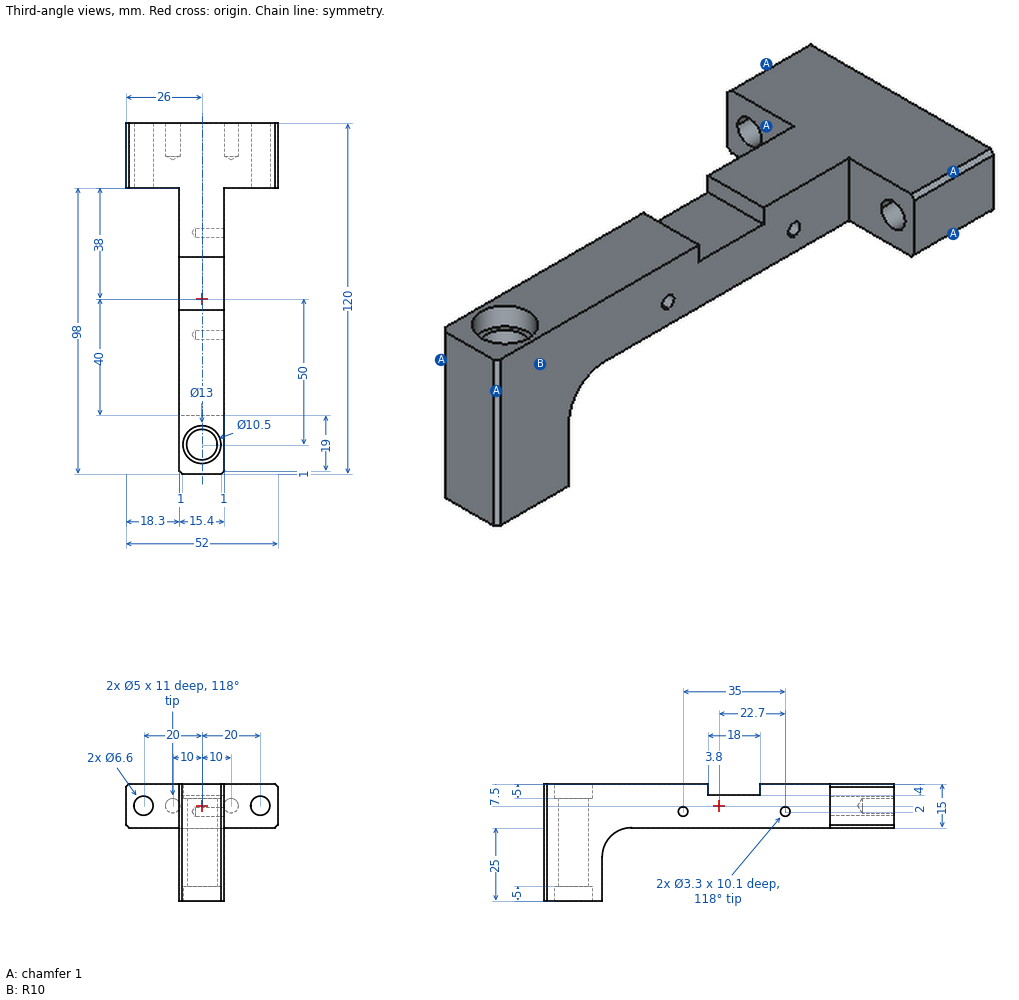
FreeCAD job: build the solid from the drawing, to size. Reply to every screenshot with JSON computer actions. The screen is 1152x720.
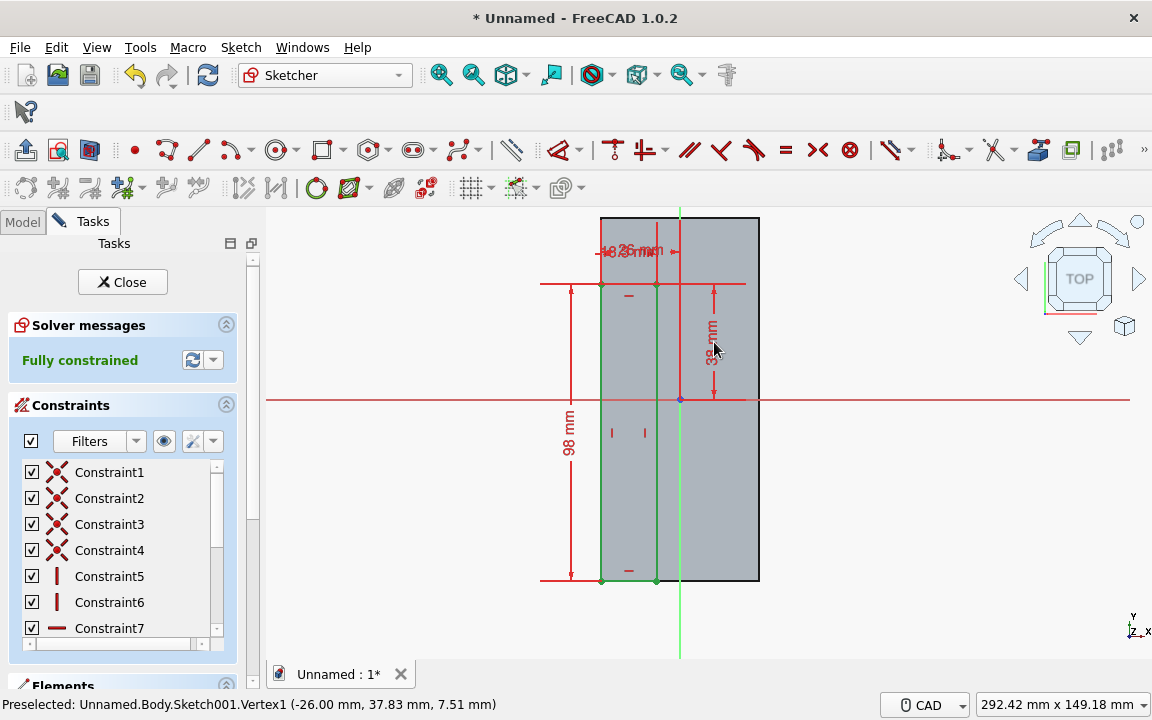
{"action": "left_click", "coordinate": [123, 282]}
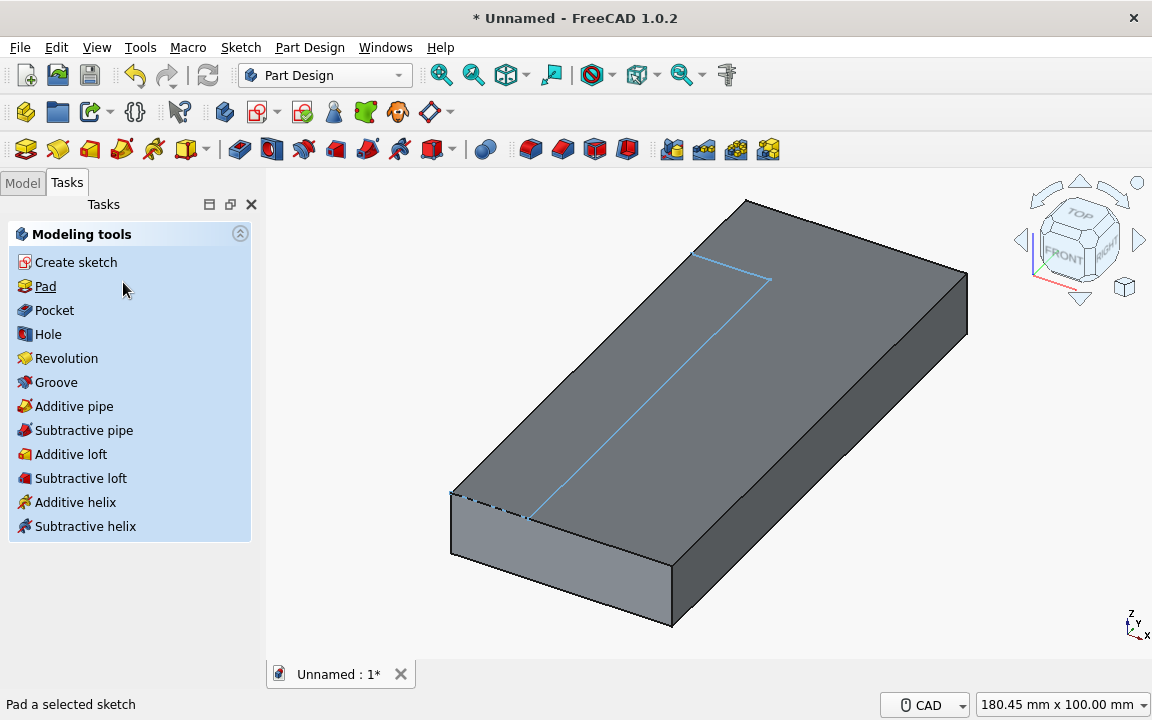
{"action": "left_click", "coordinate": [240, 150]}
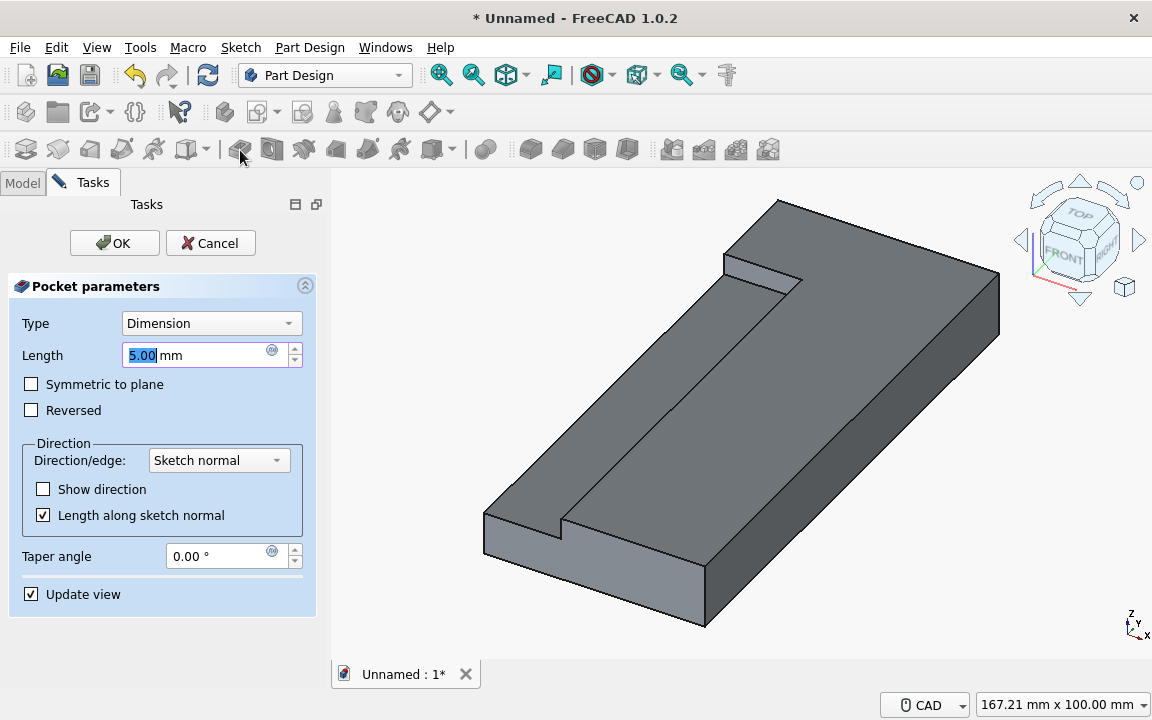
{"action": "left_click", "coordinate": [212, 324]}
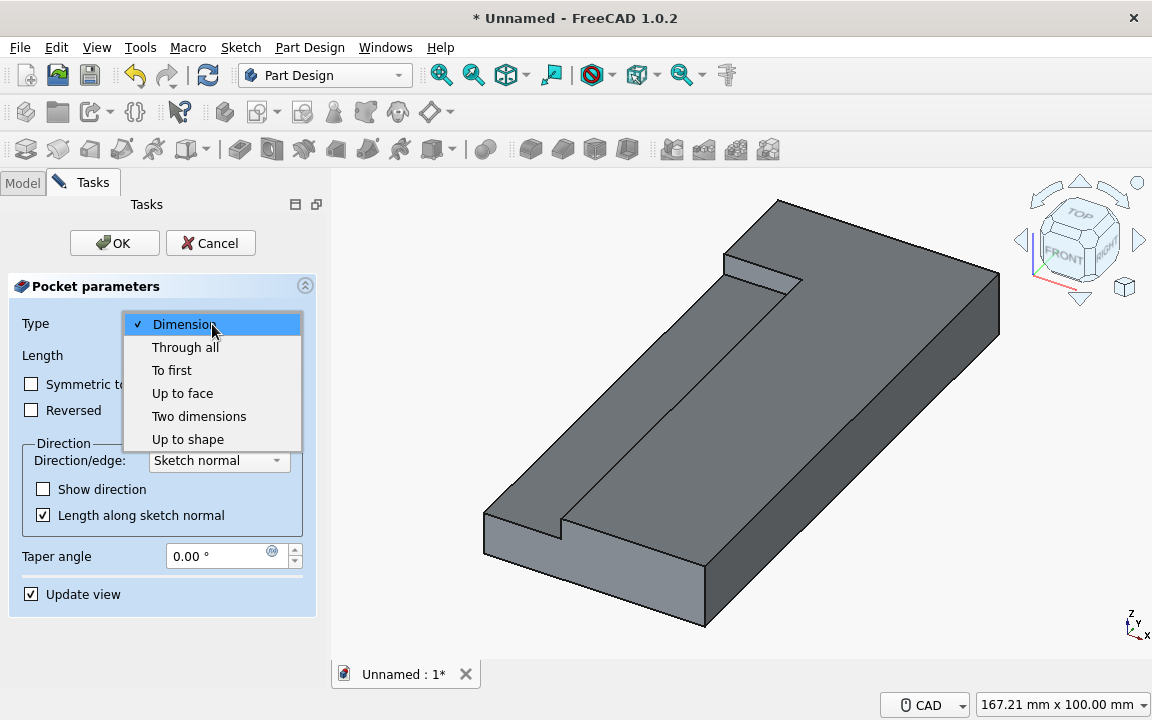
{"action": "left_click", "coordinate": [212, 348]}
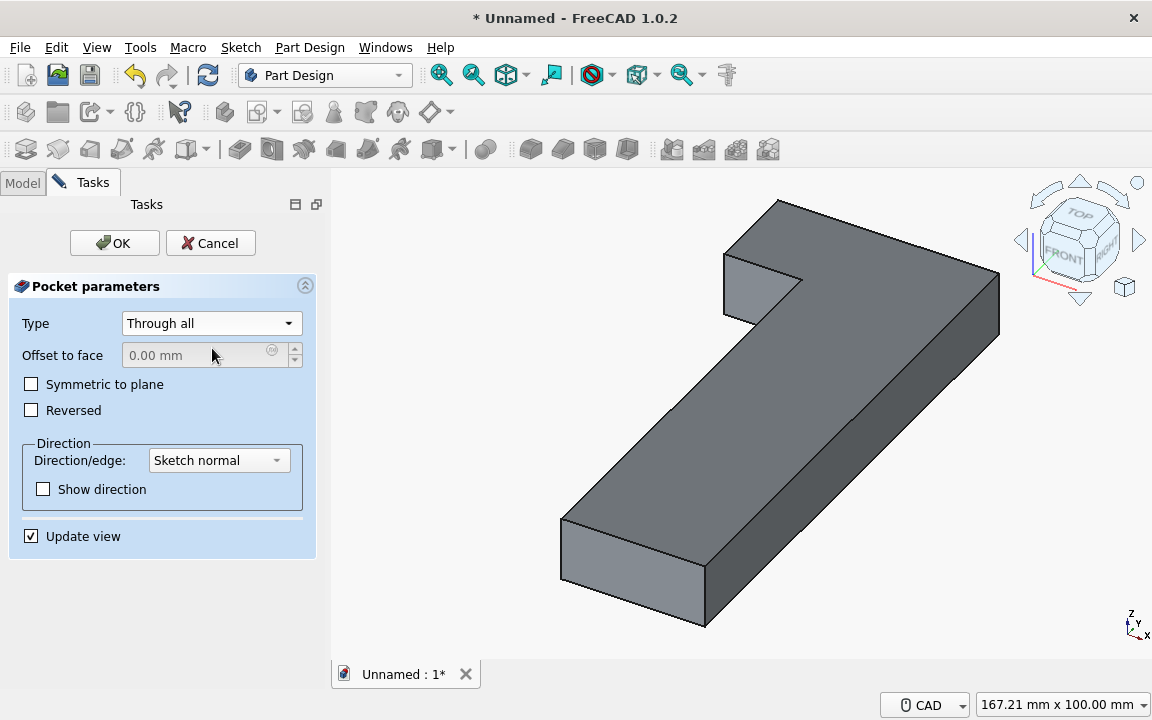
{"action": "left_click", "coordinate": [115, 243]}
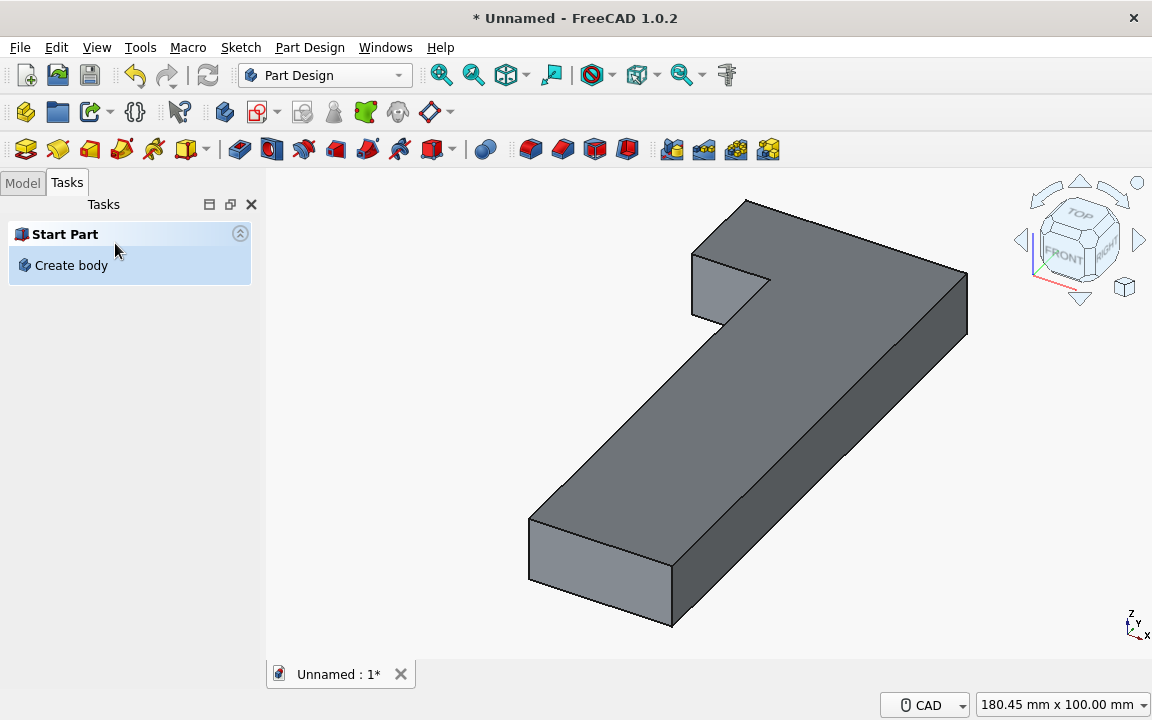
{"action": "left_click", "coordinate": [23, 182]}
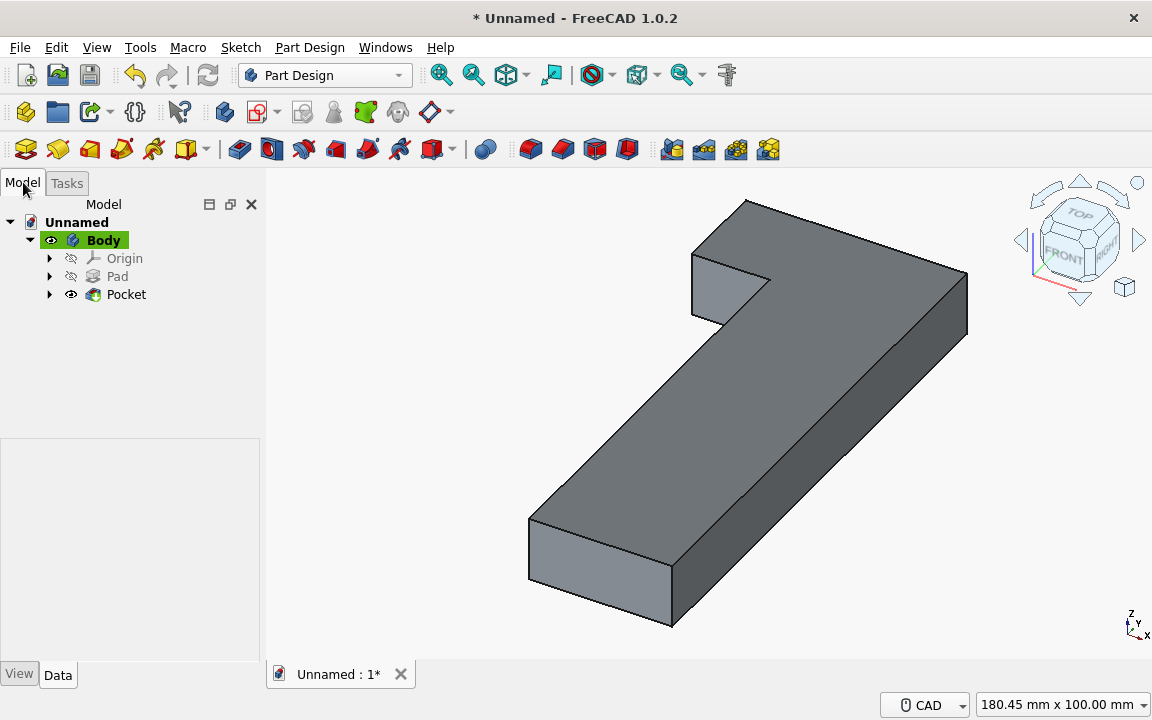
{"action": "left_click", "coordinate": [116, 294]}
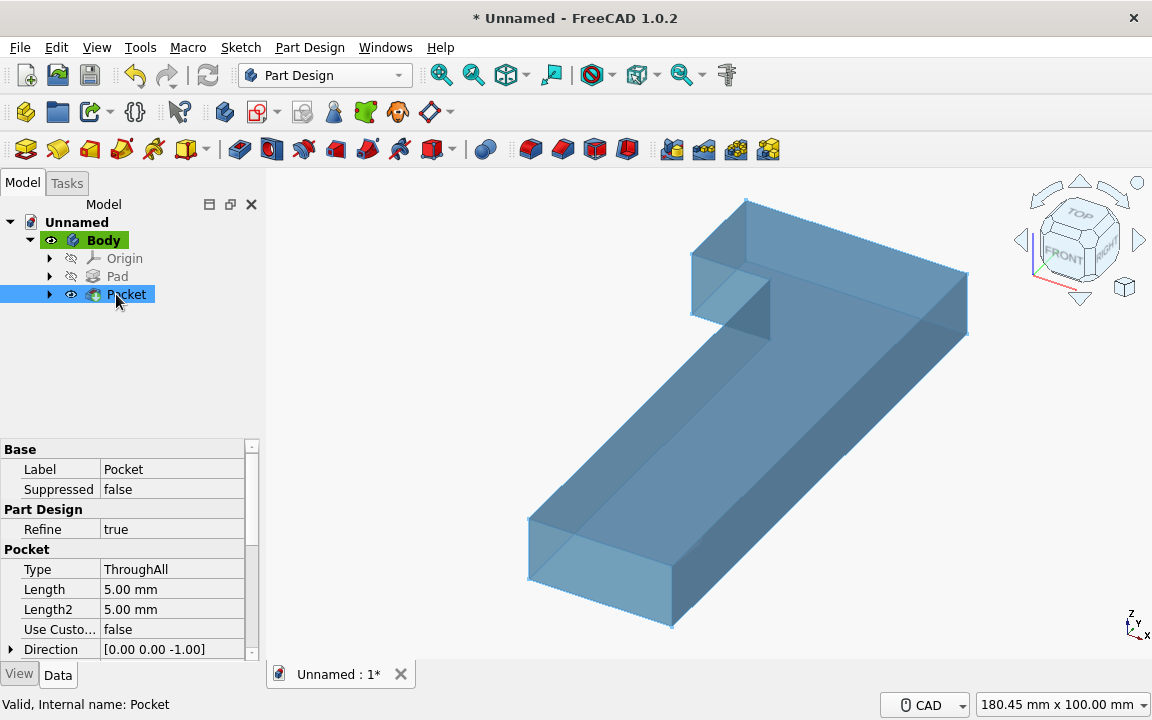
{"action": "left_click", "coordinate": [672, 150]}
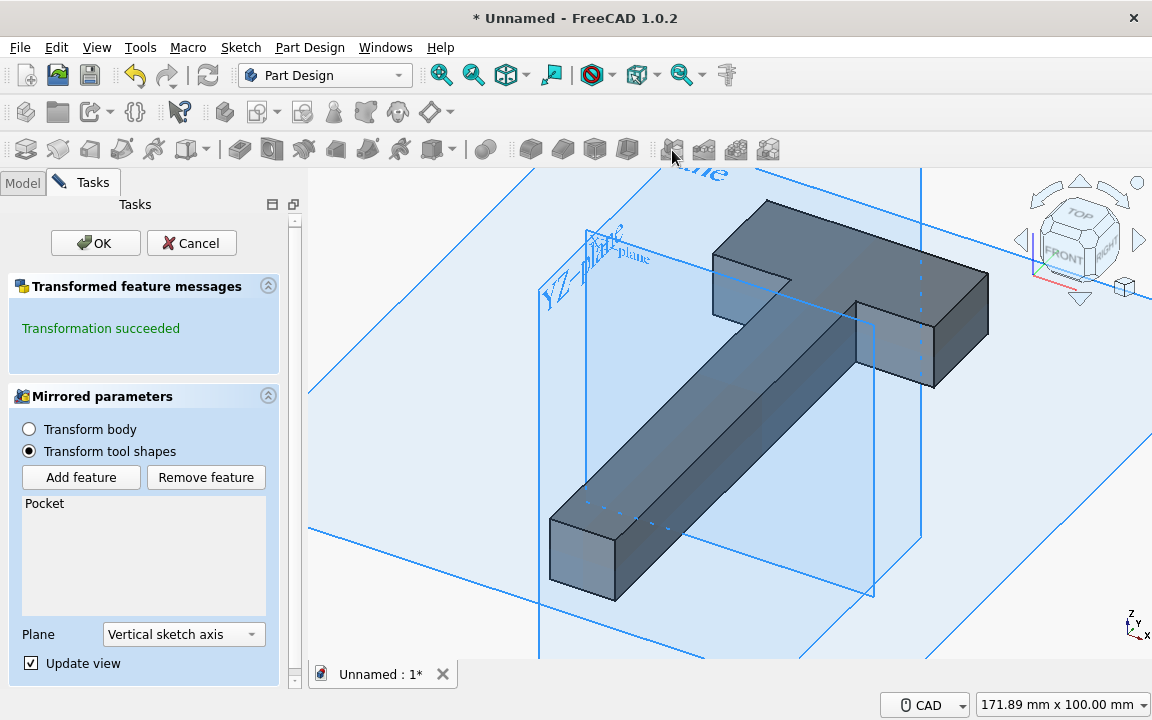
{"action": "left_click", "coordinate": [184, 634]}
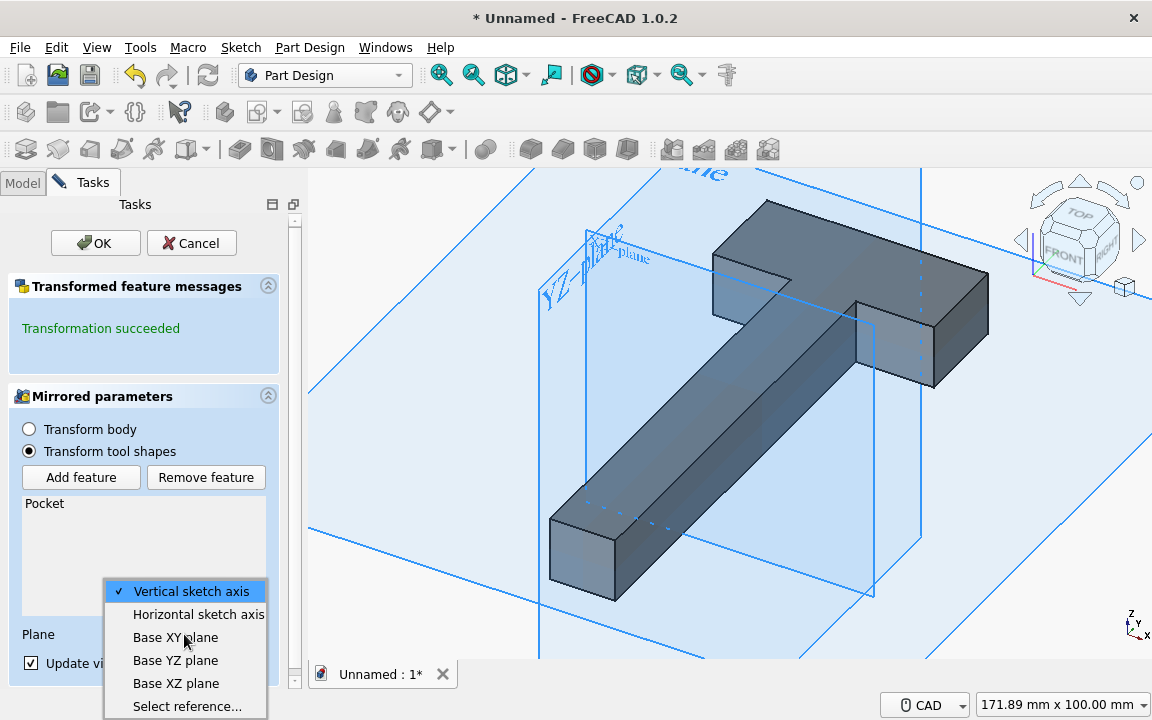
{"action": "left_click", "coordinate": [184, 660]}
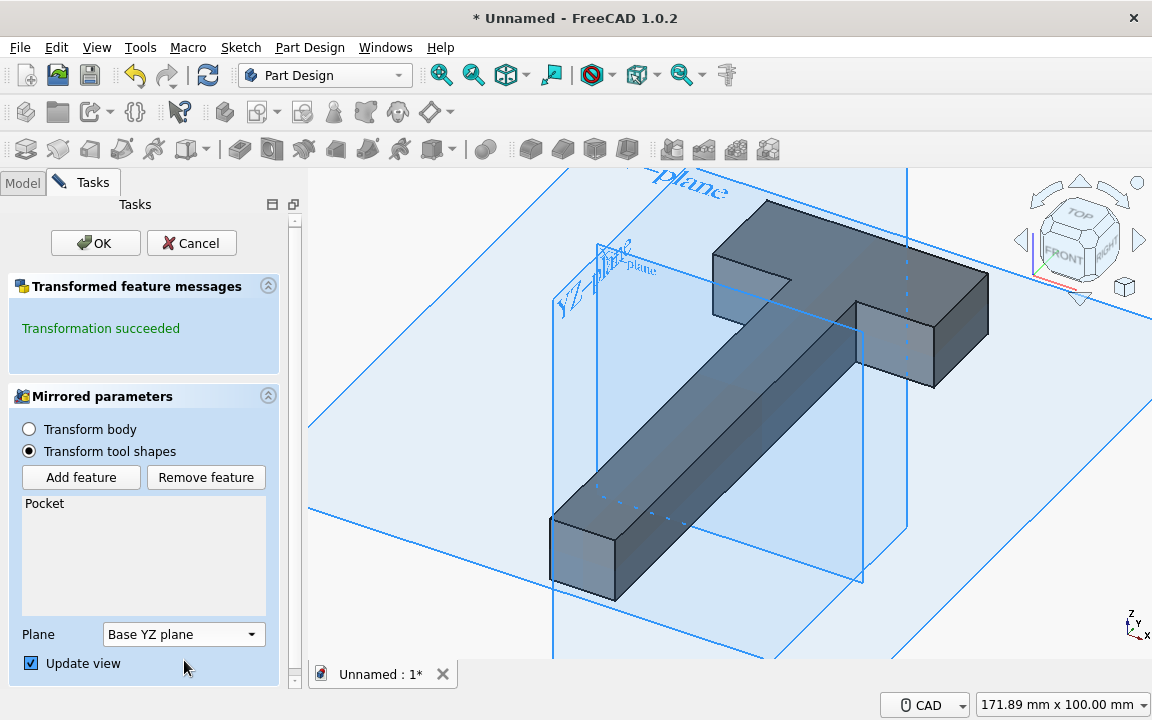
{"action": "left_click", "coordinate": [96, 243]}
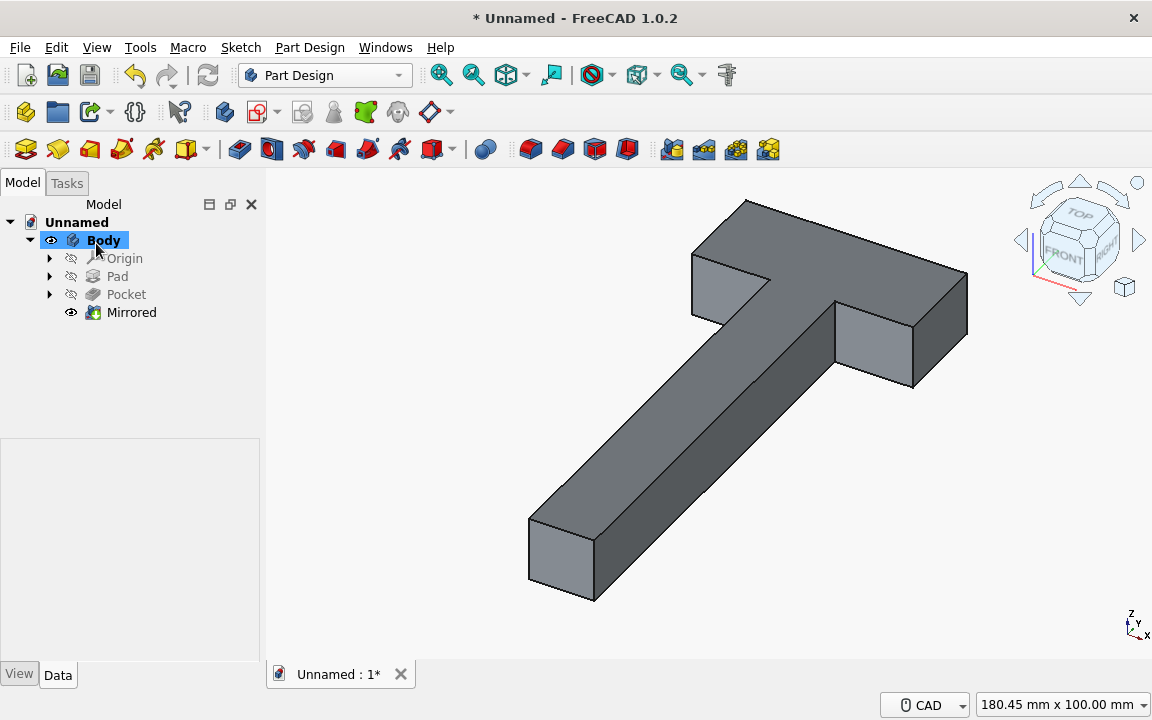
{"action": "key", "text": "4"}